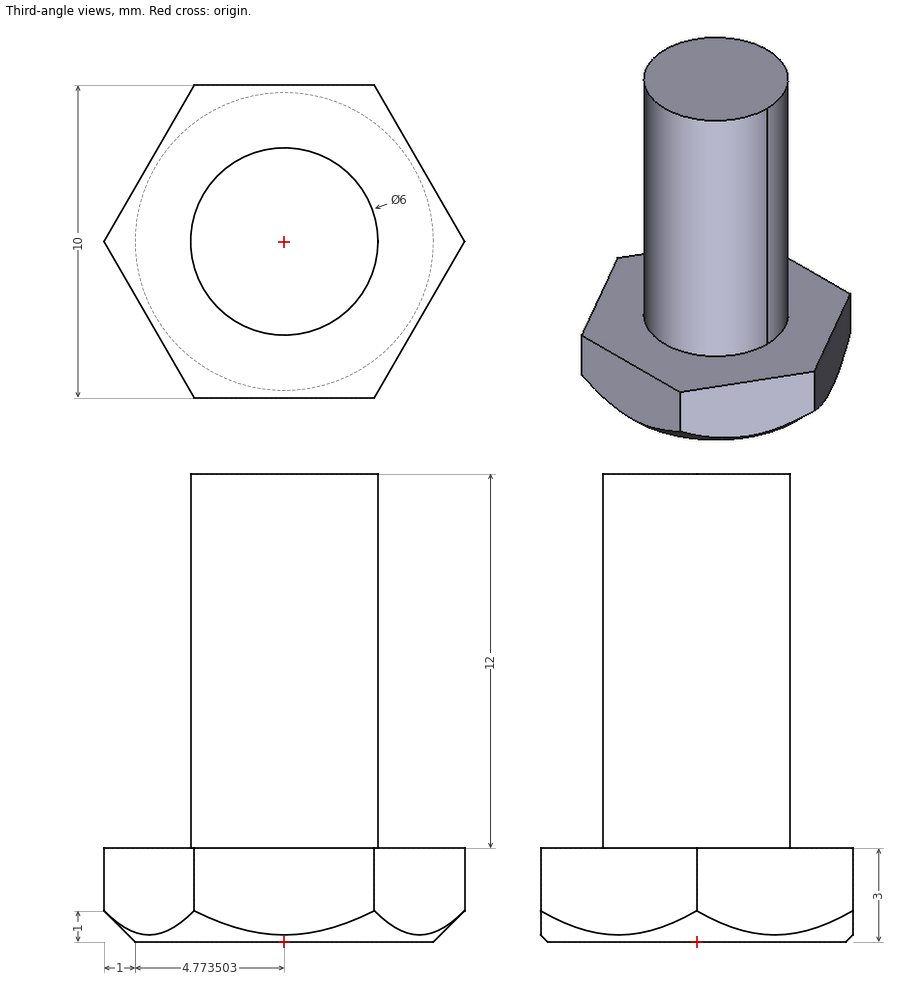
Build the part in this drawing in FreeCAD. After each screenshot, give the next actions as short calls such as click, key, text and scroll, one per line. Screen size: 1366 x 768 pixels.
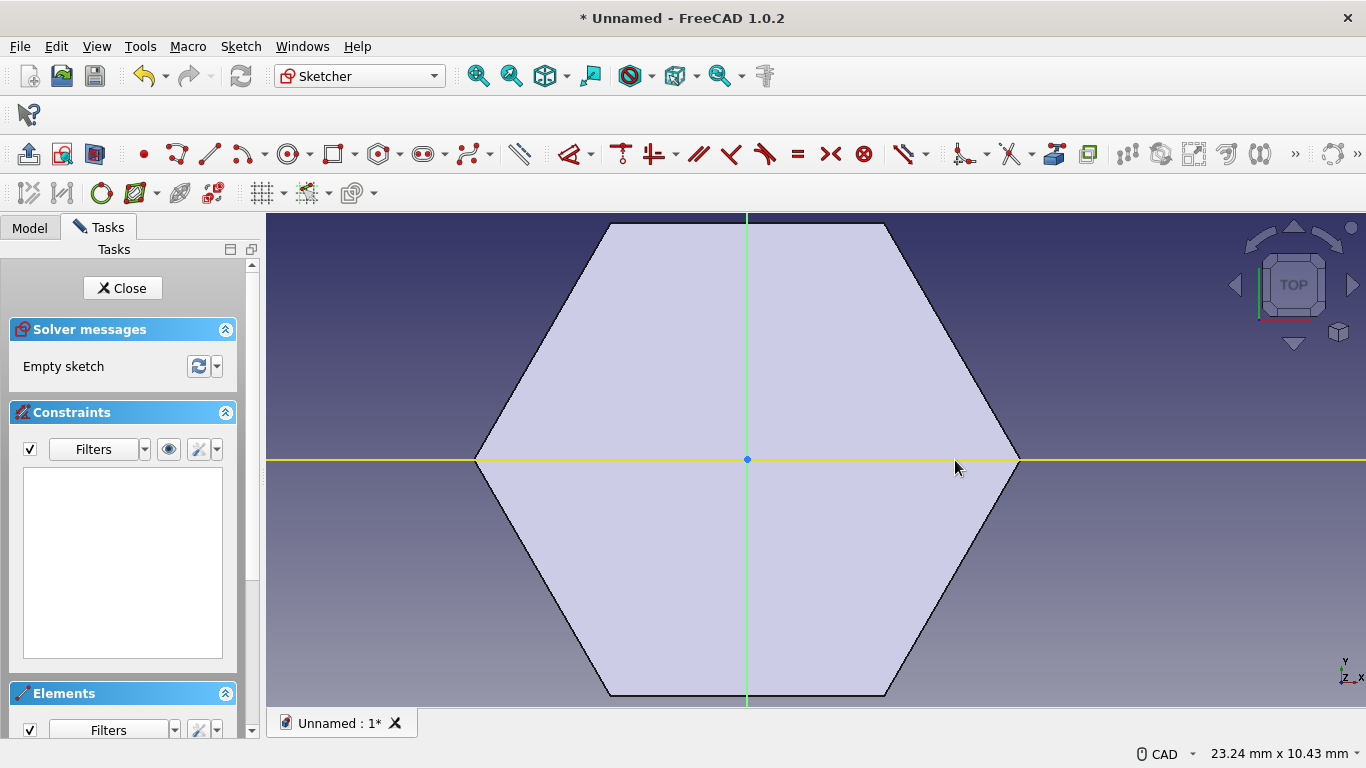
click(288, 154)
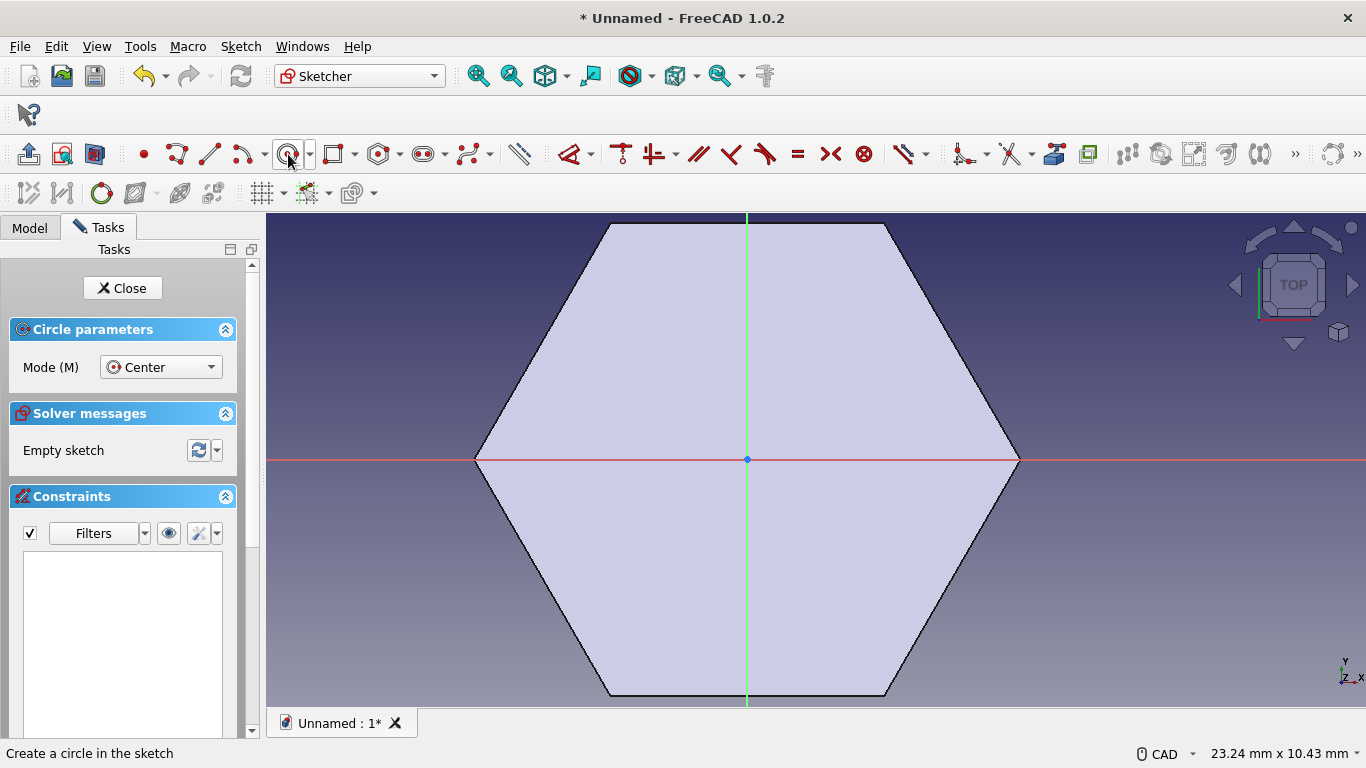
click(747, 460)
move(848, 359)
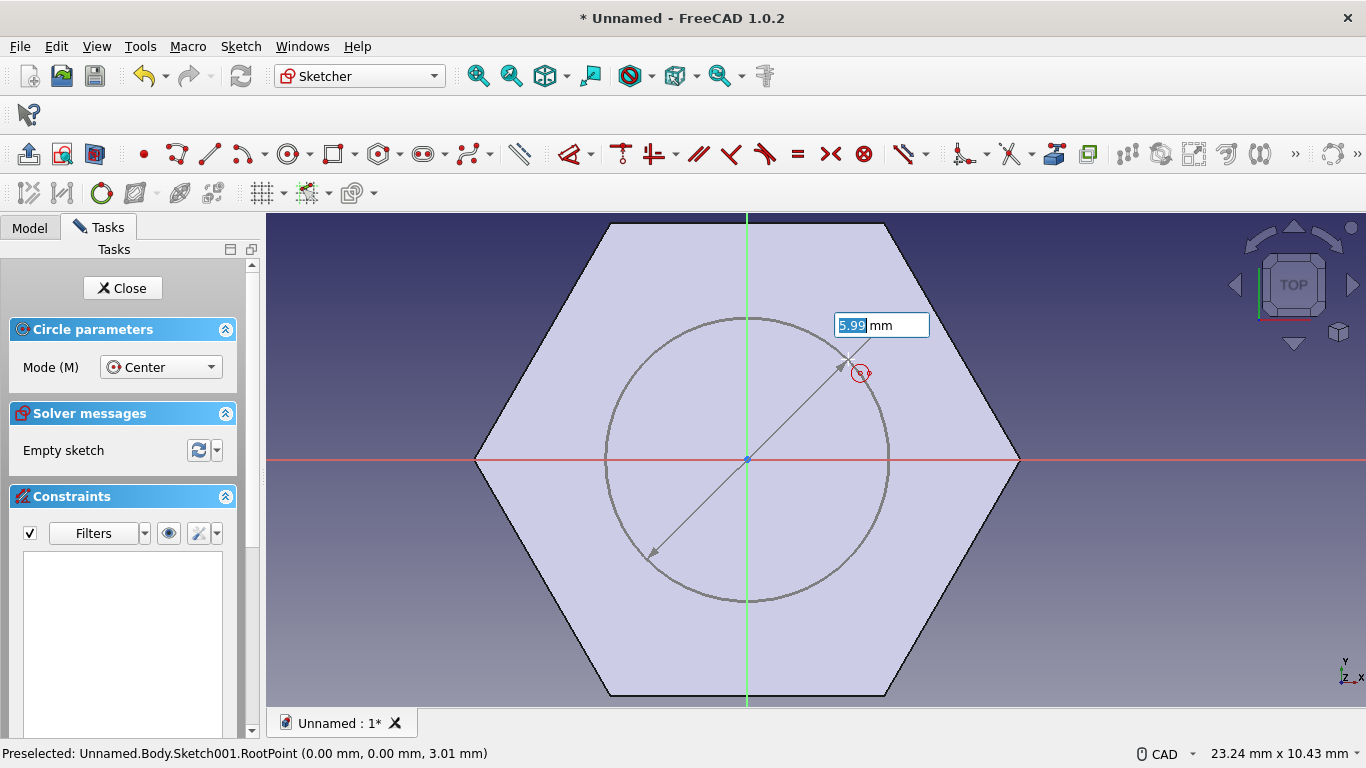
text(6)
key(Return)
key(Escape)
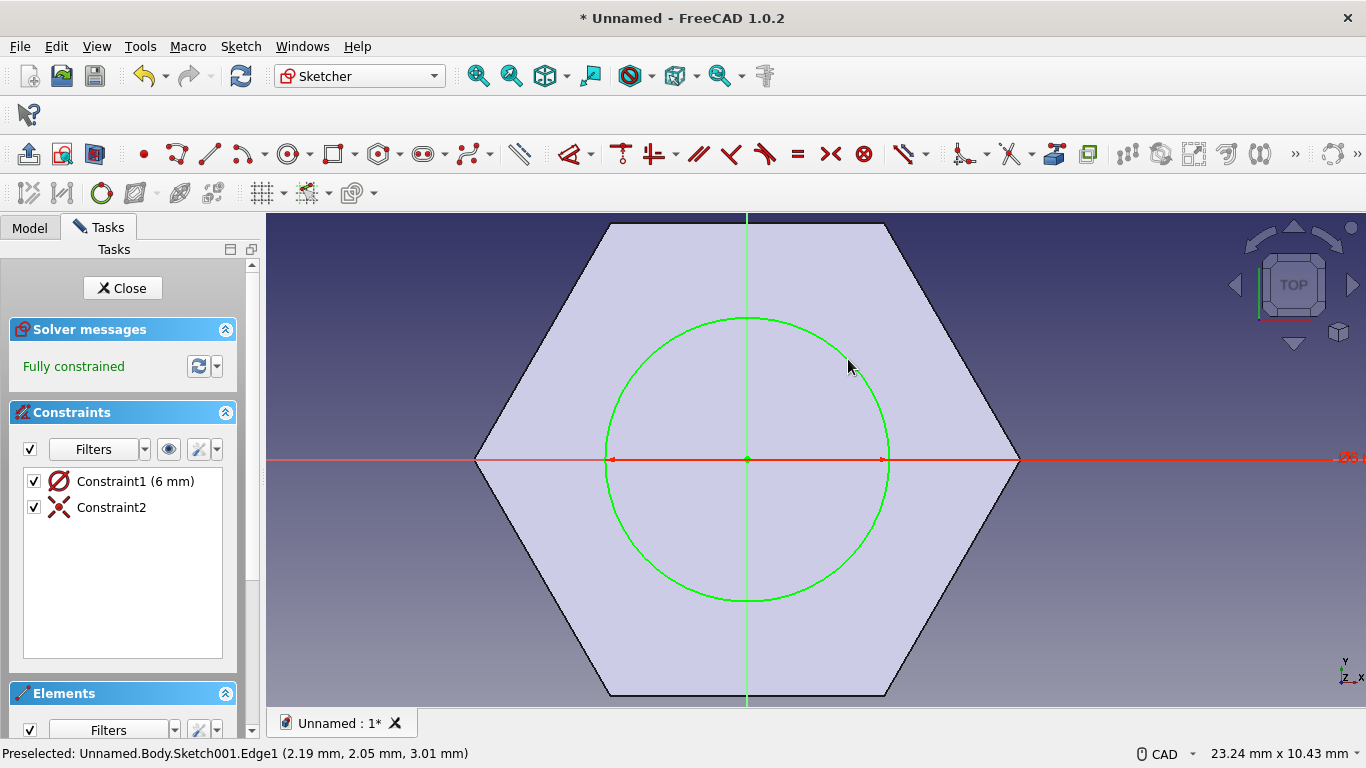
click(123, 288)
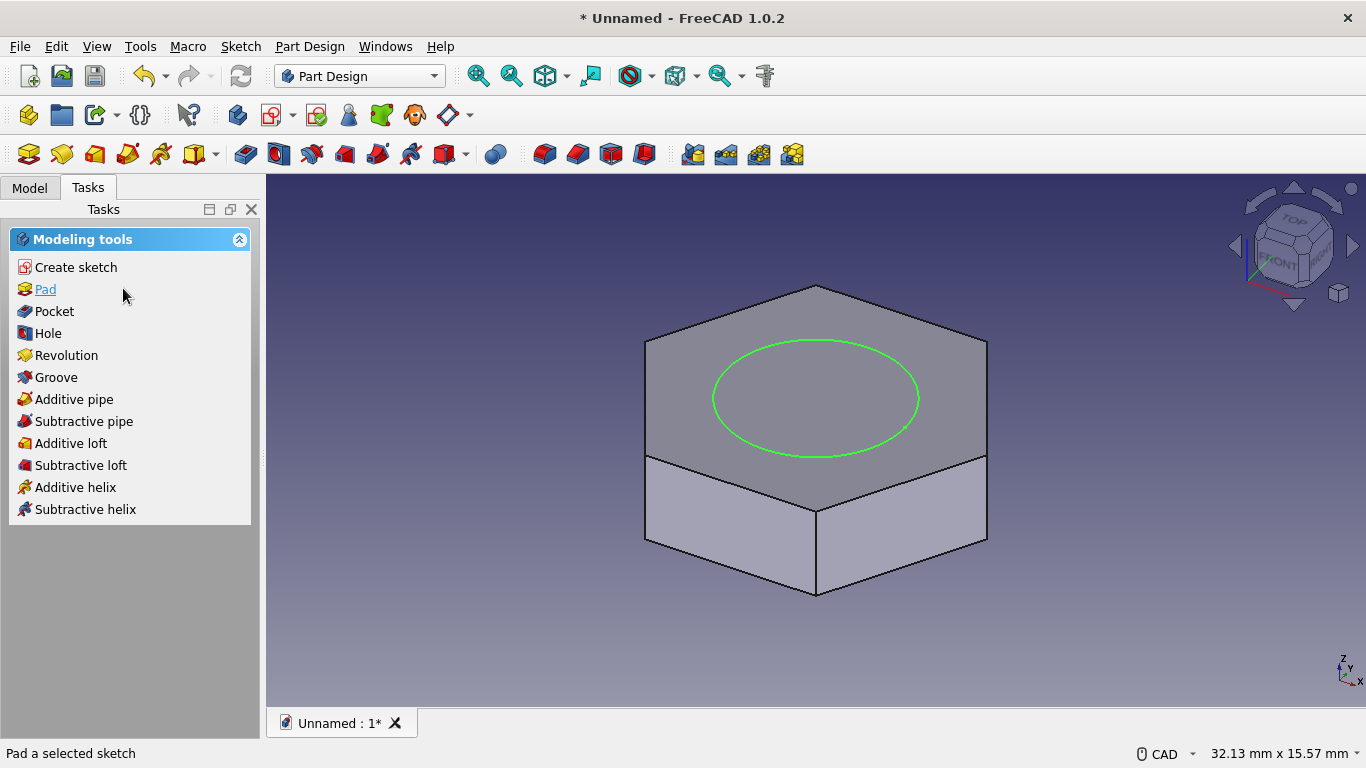
click(29, 154)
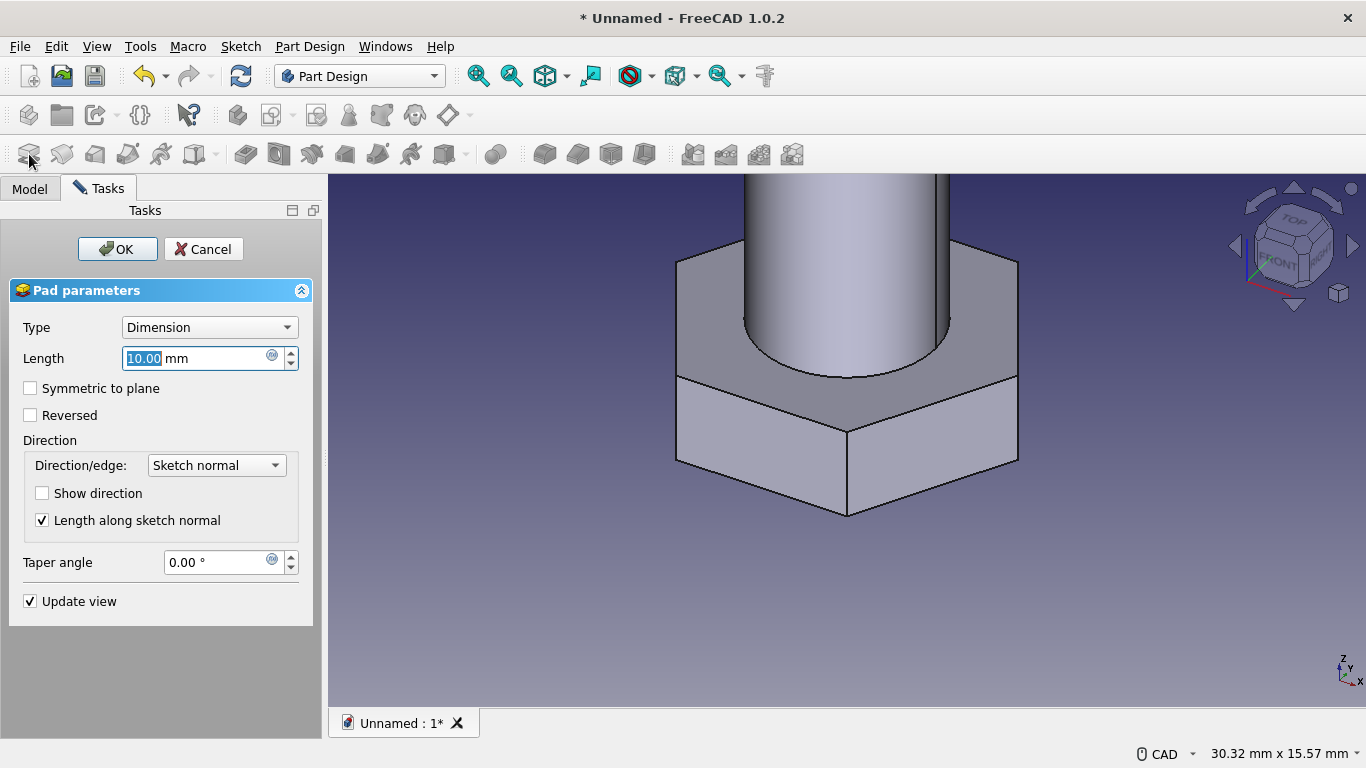
text(12)
key(Tab)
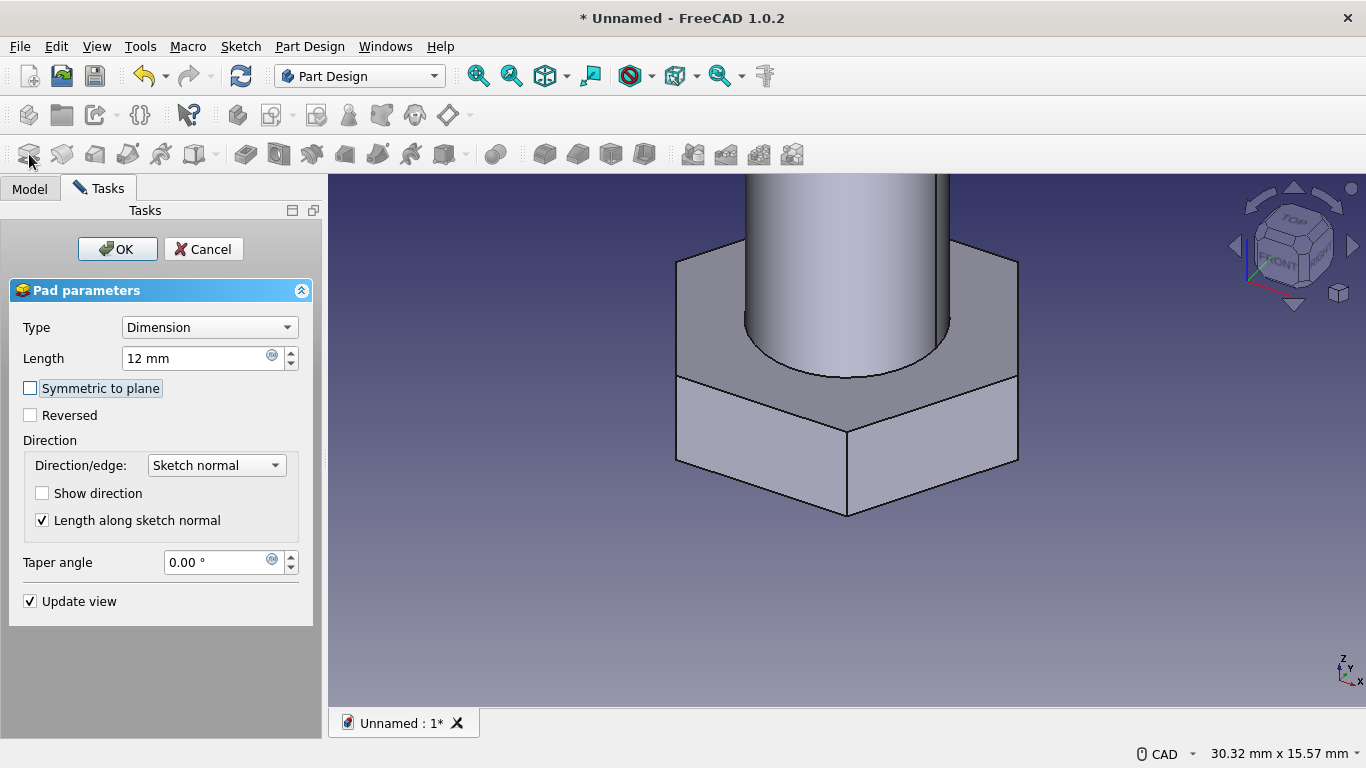
click(118, 249)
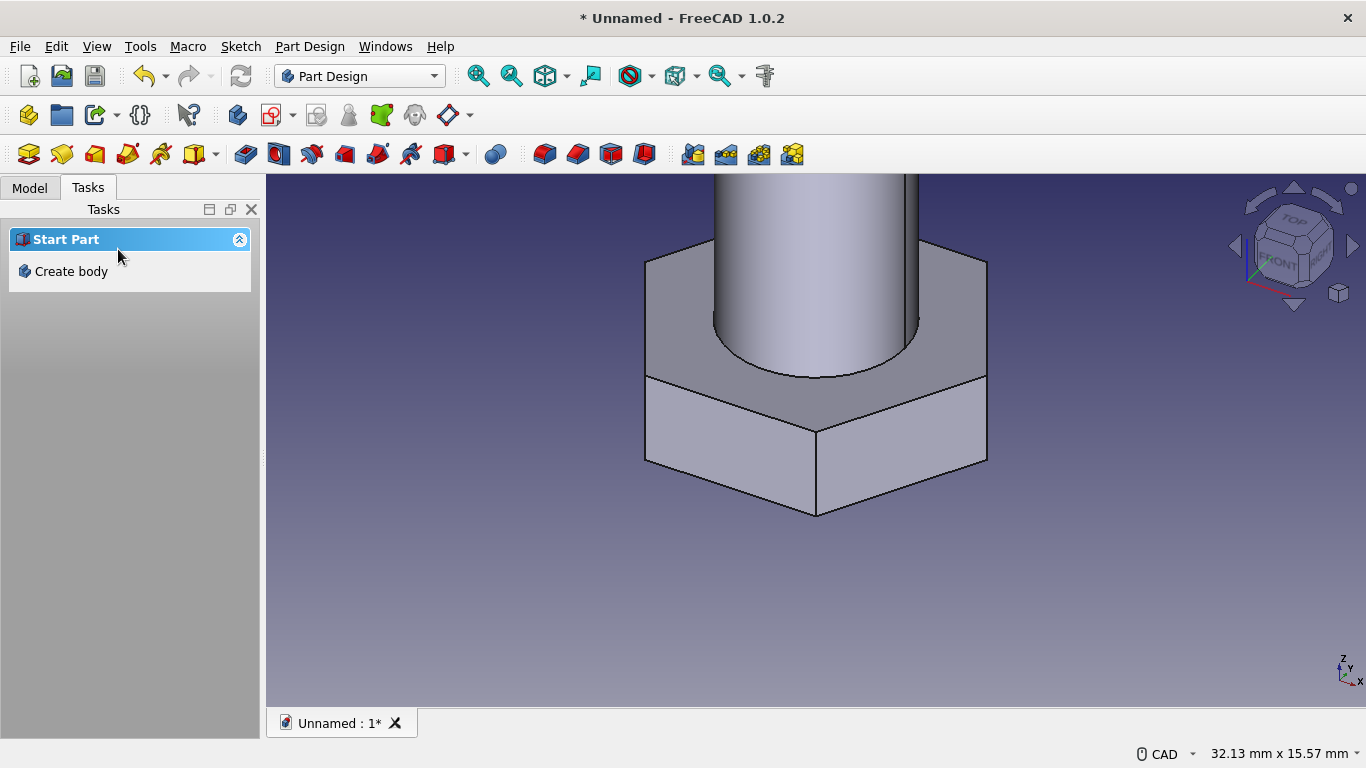
click(479, 76)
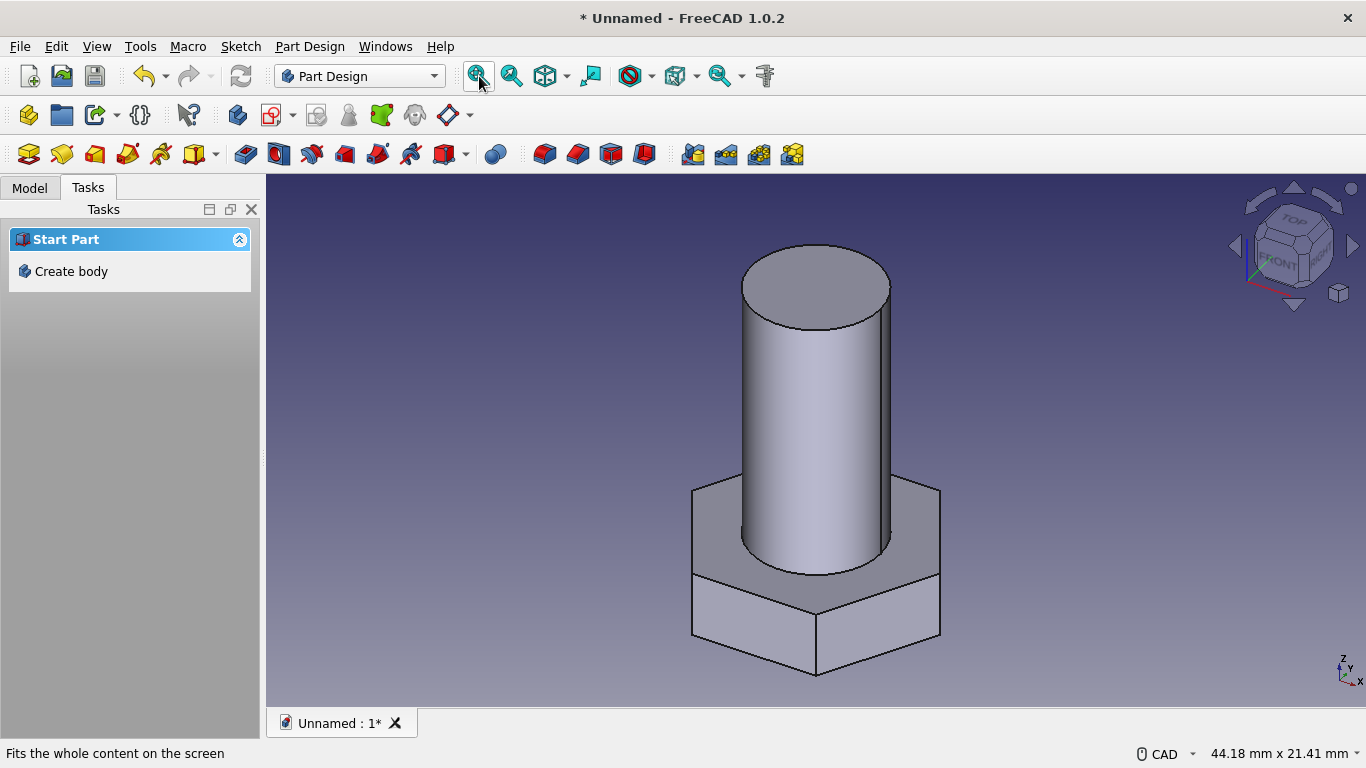
click(270, 116)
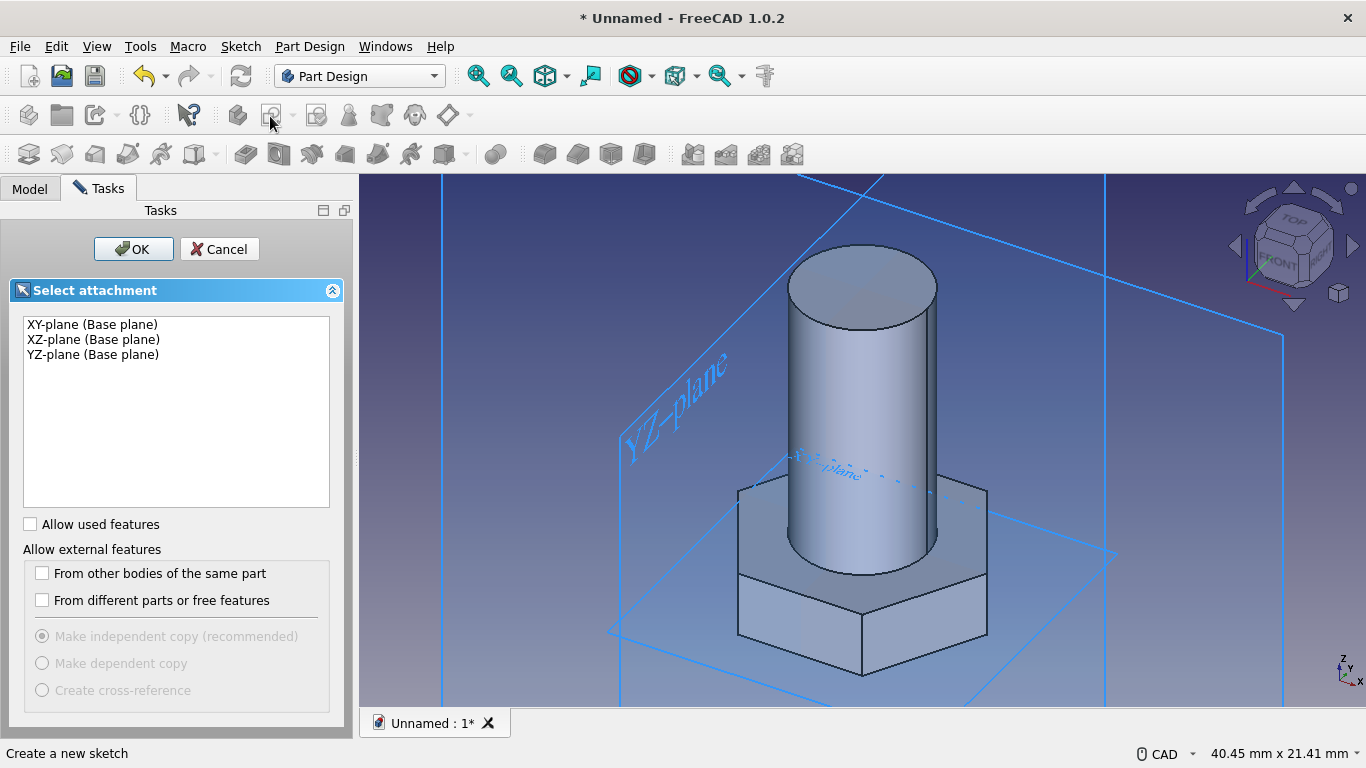
click(84, 340)